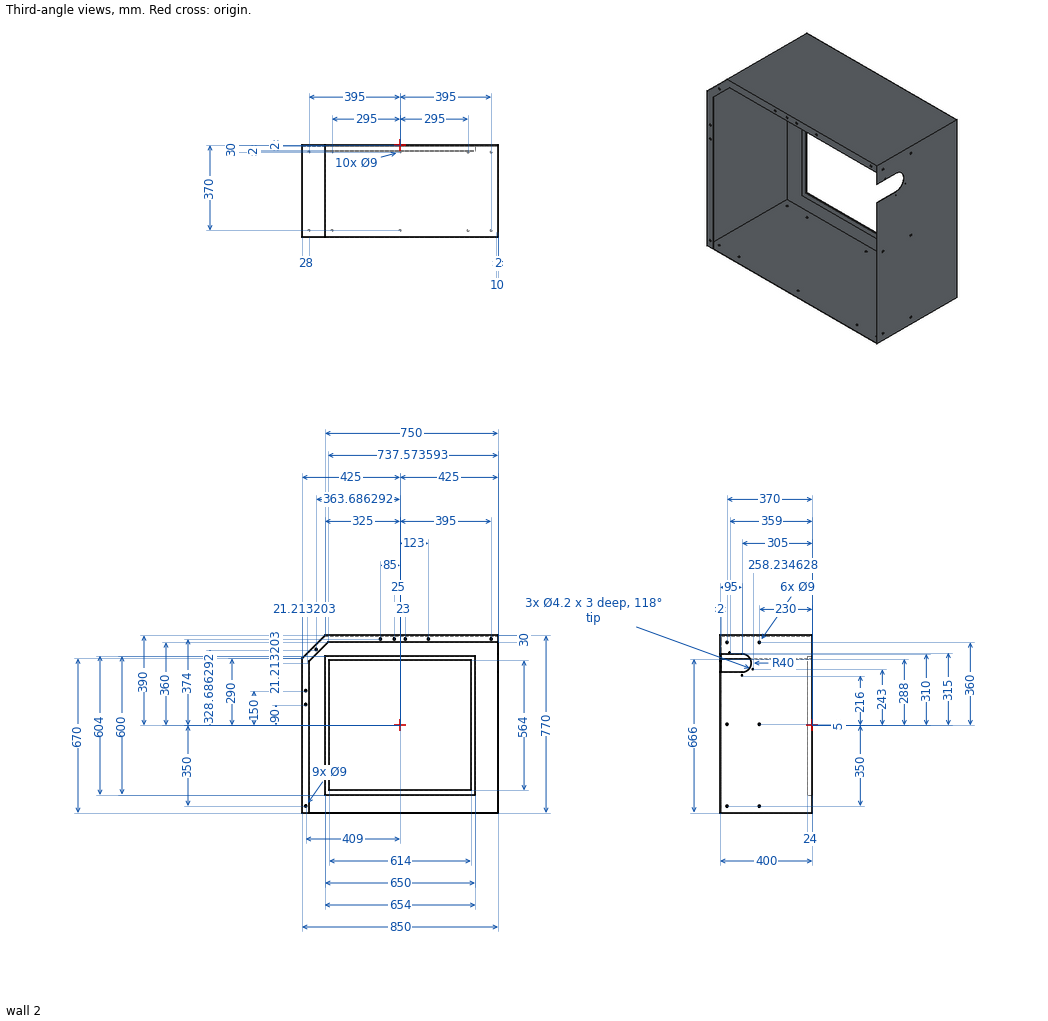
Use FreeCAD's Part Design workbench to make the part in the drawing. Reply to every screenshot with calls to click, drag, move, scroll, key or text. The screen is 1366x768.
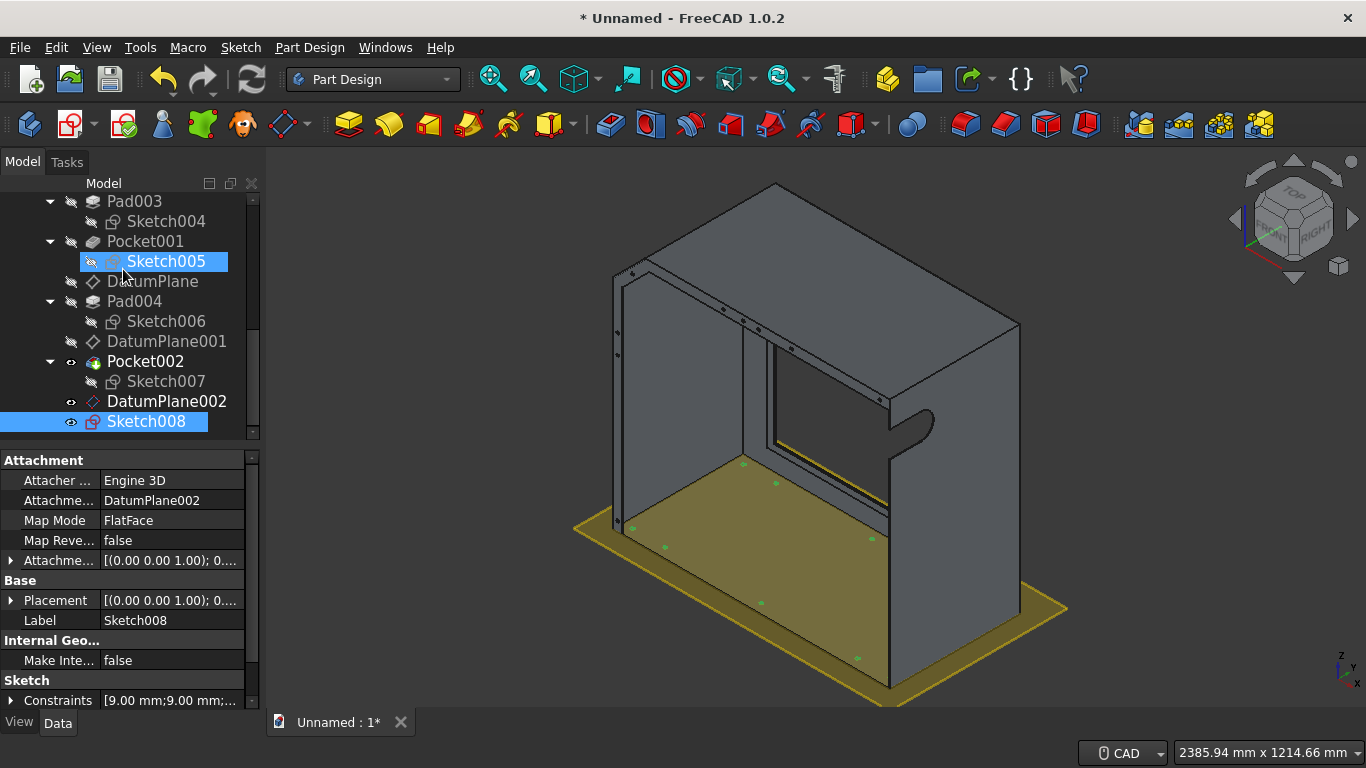
click(612, 124)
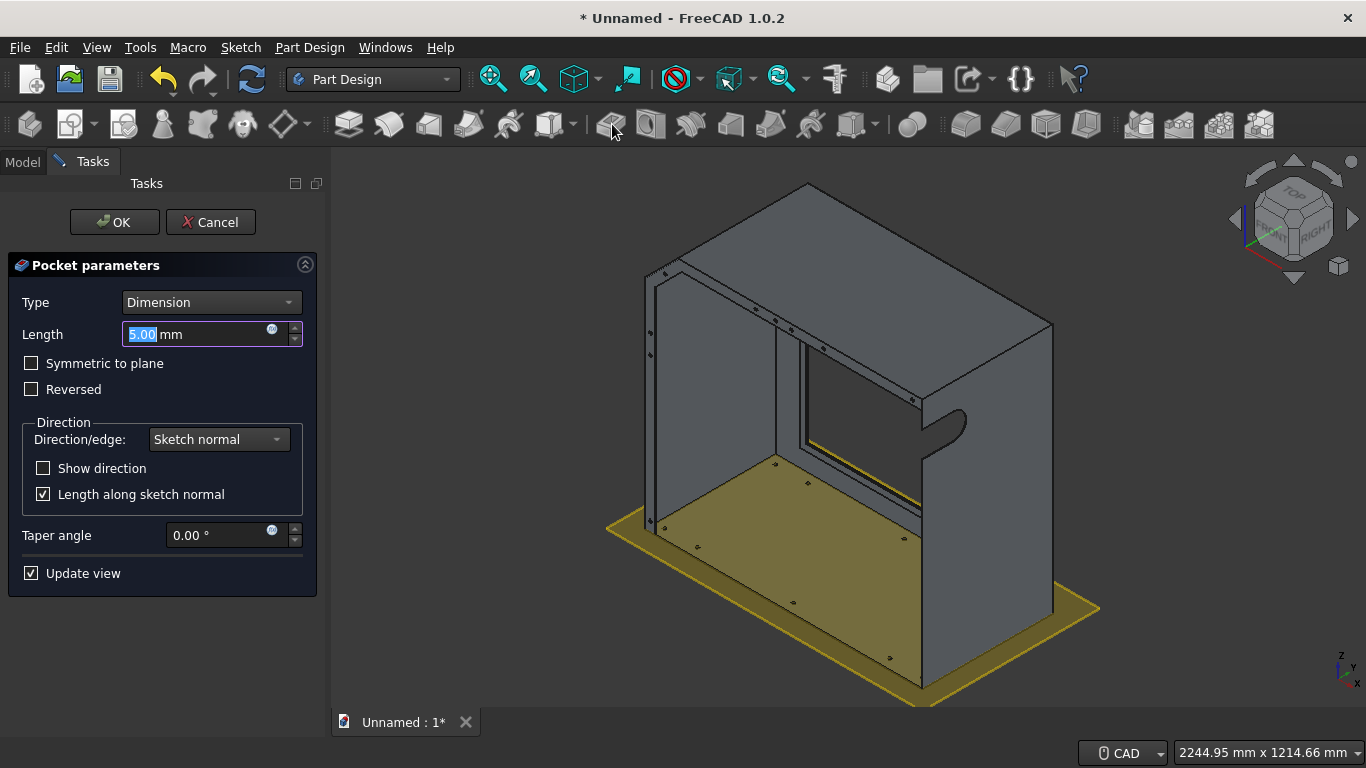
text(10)
key(Tab)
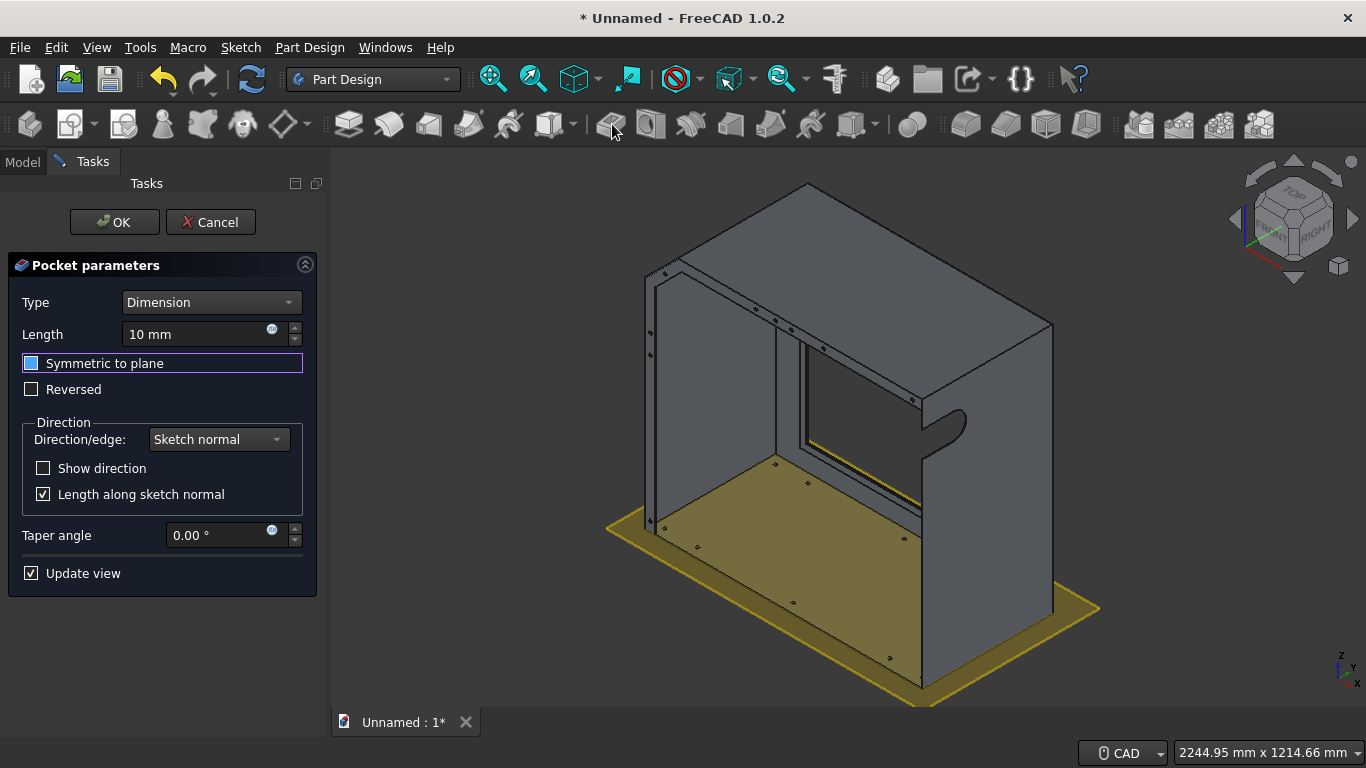
click(115, 222)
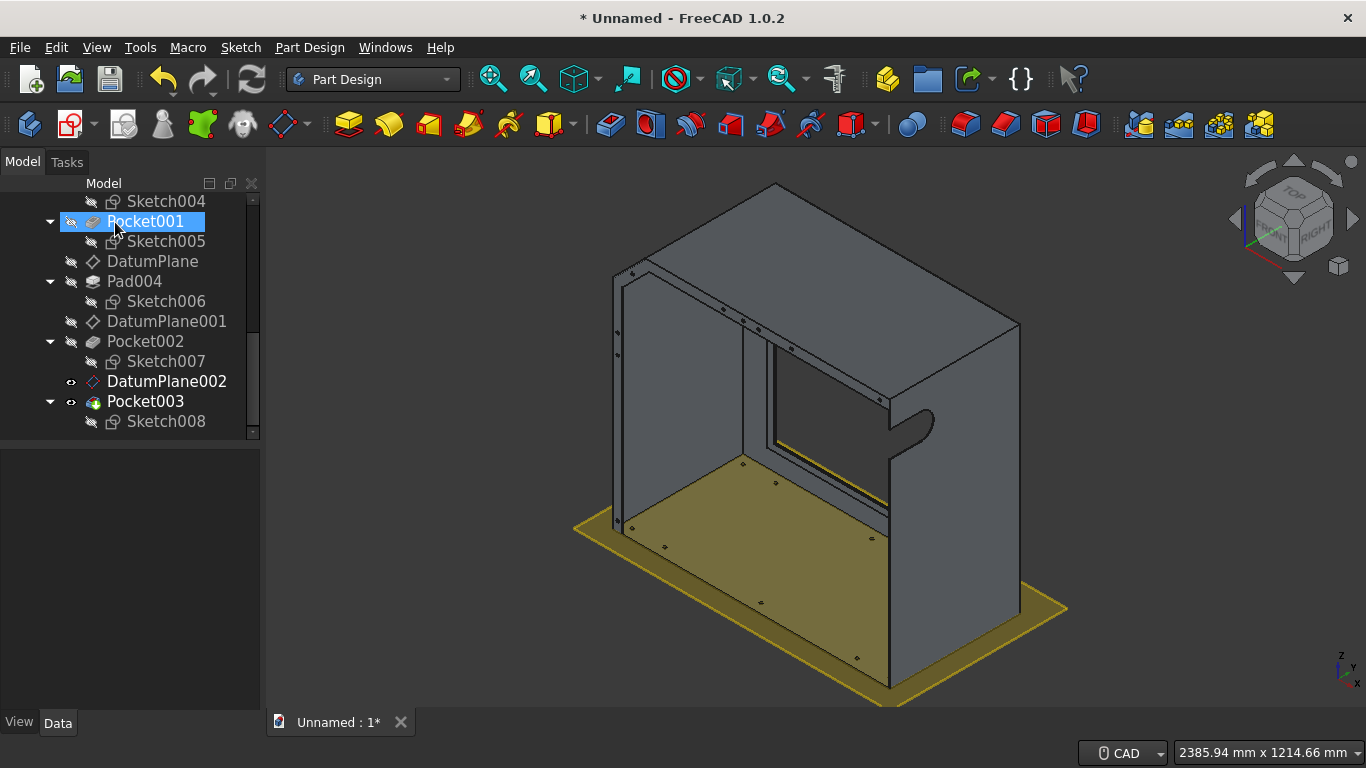
click(116, 382)
key(space)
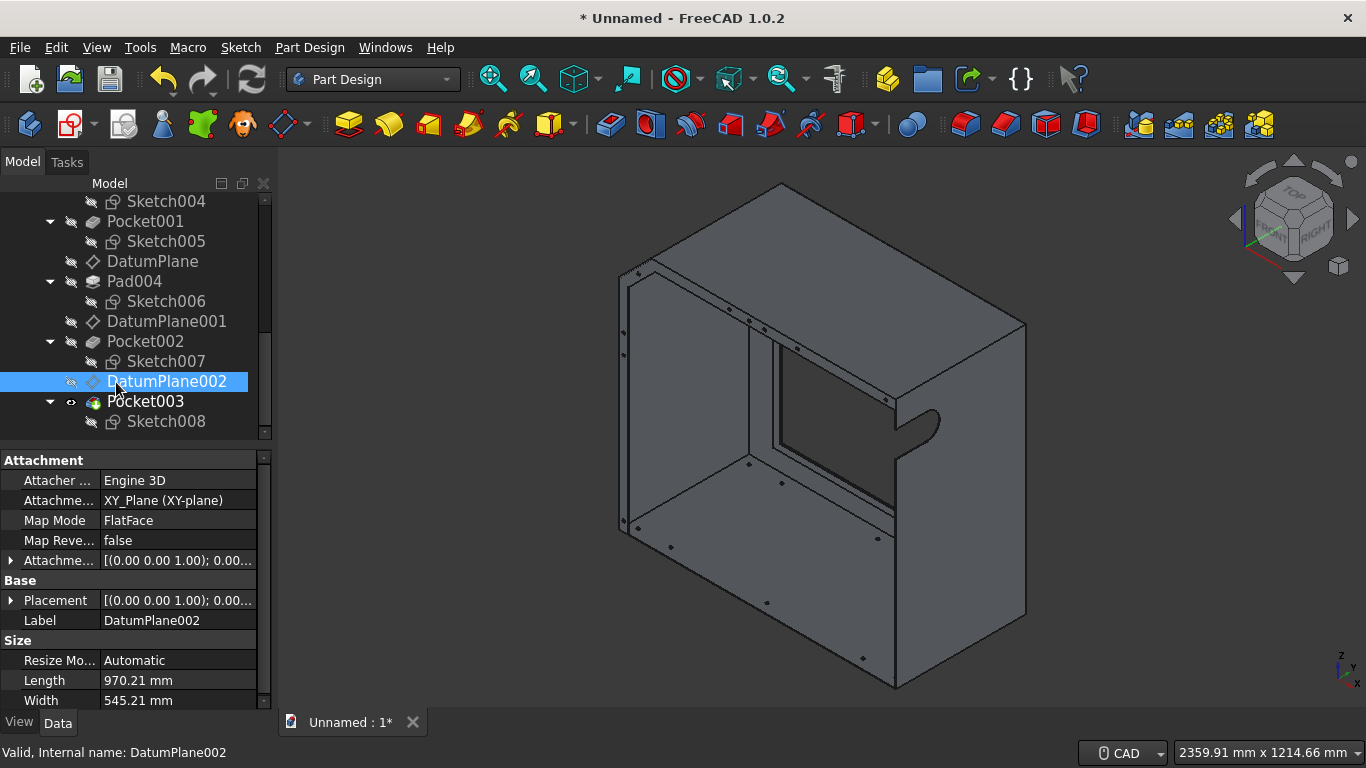
click(961, 506)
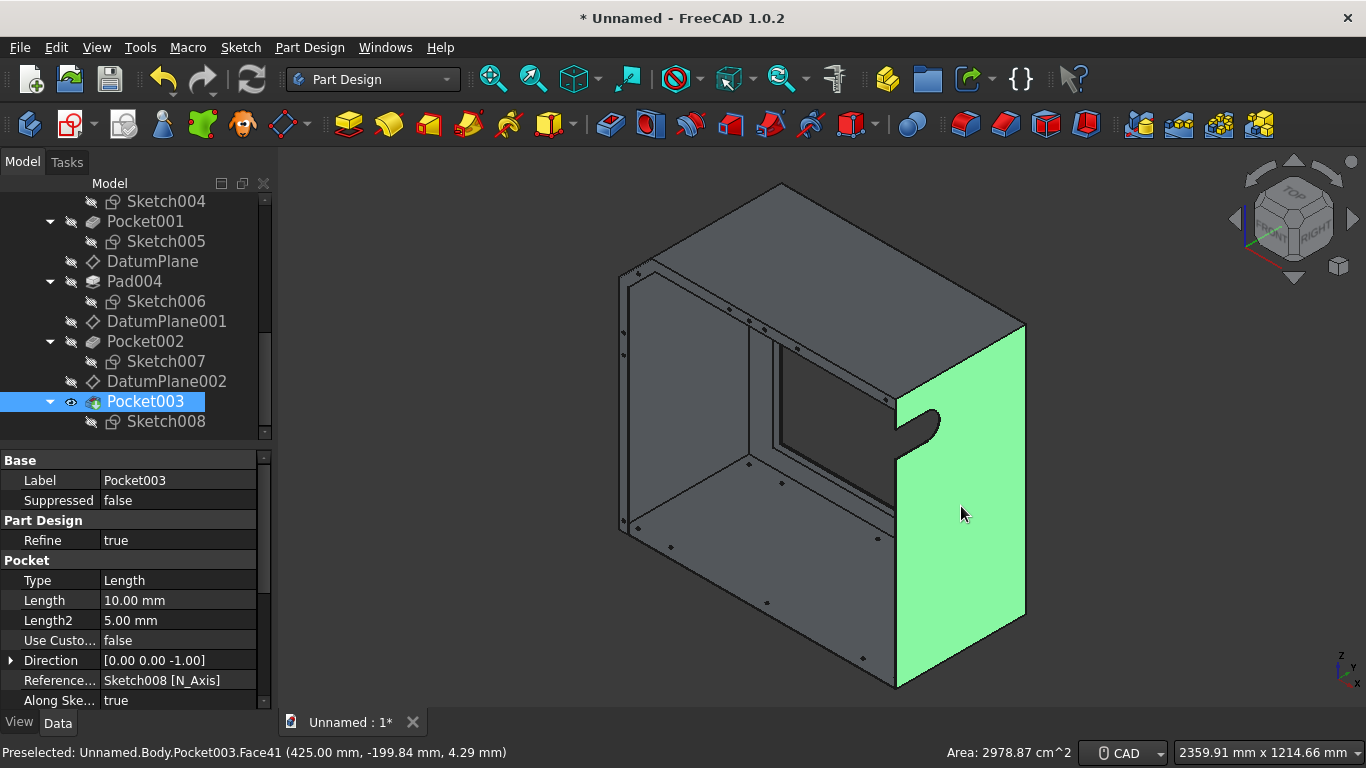
click(70, 124)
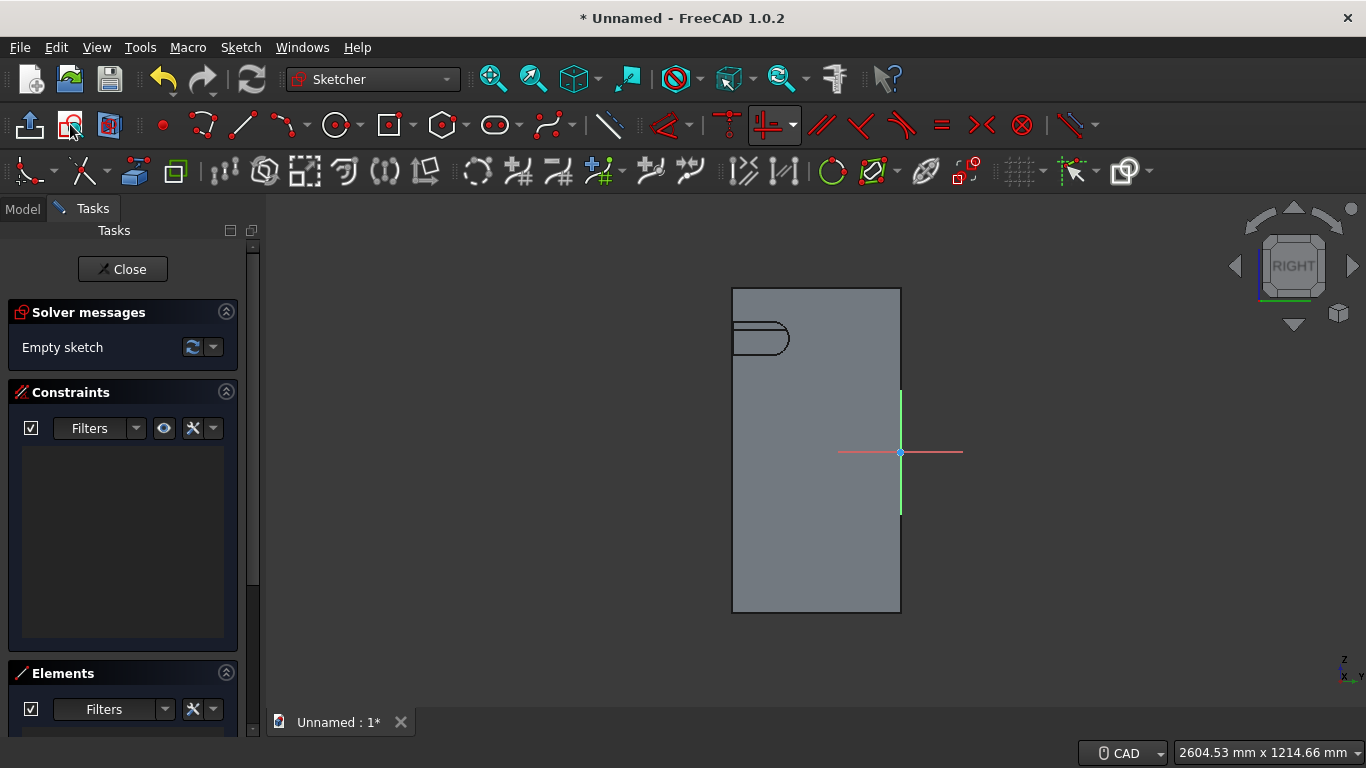
click(336, 126)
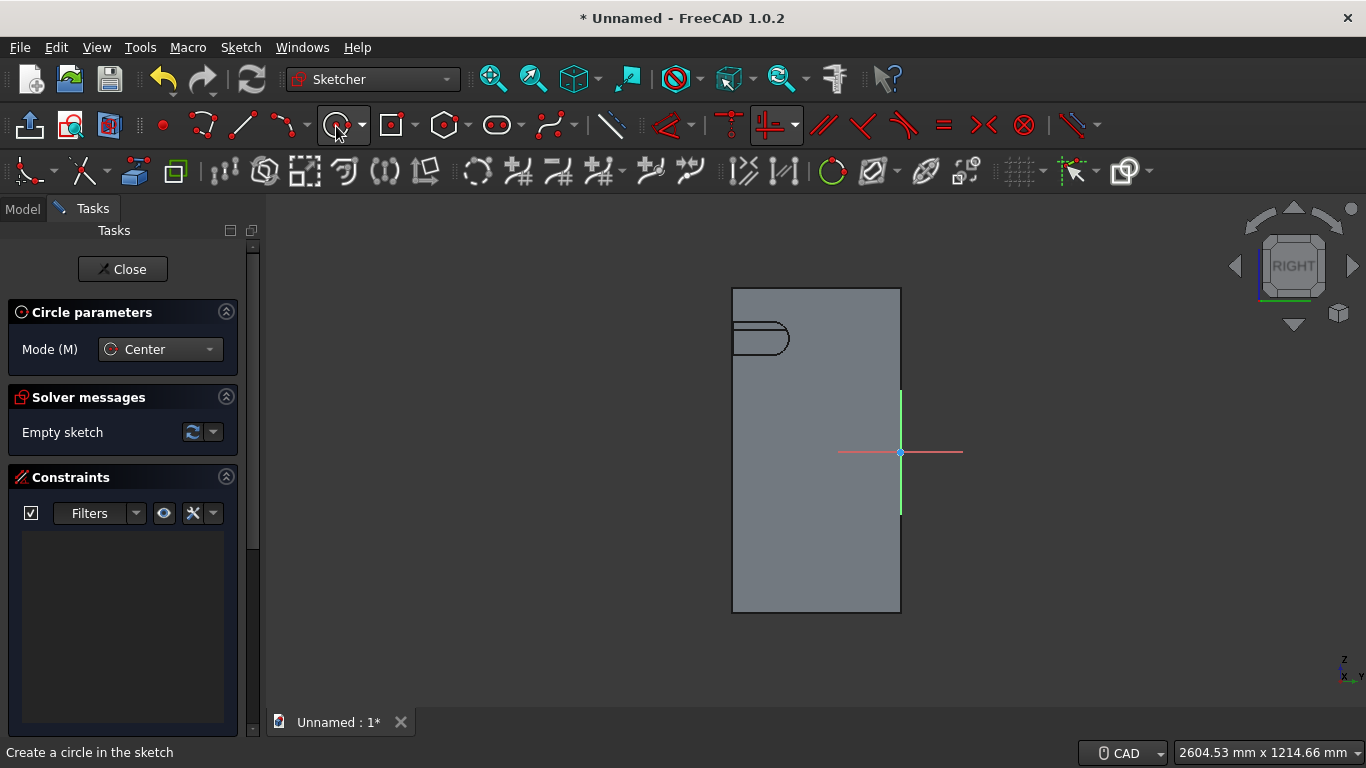
scroll(804, 300, up, 13)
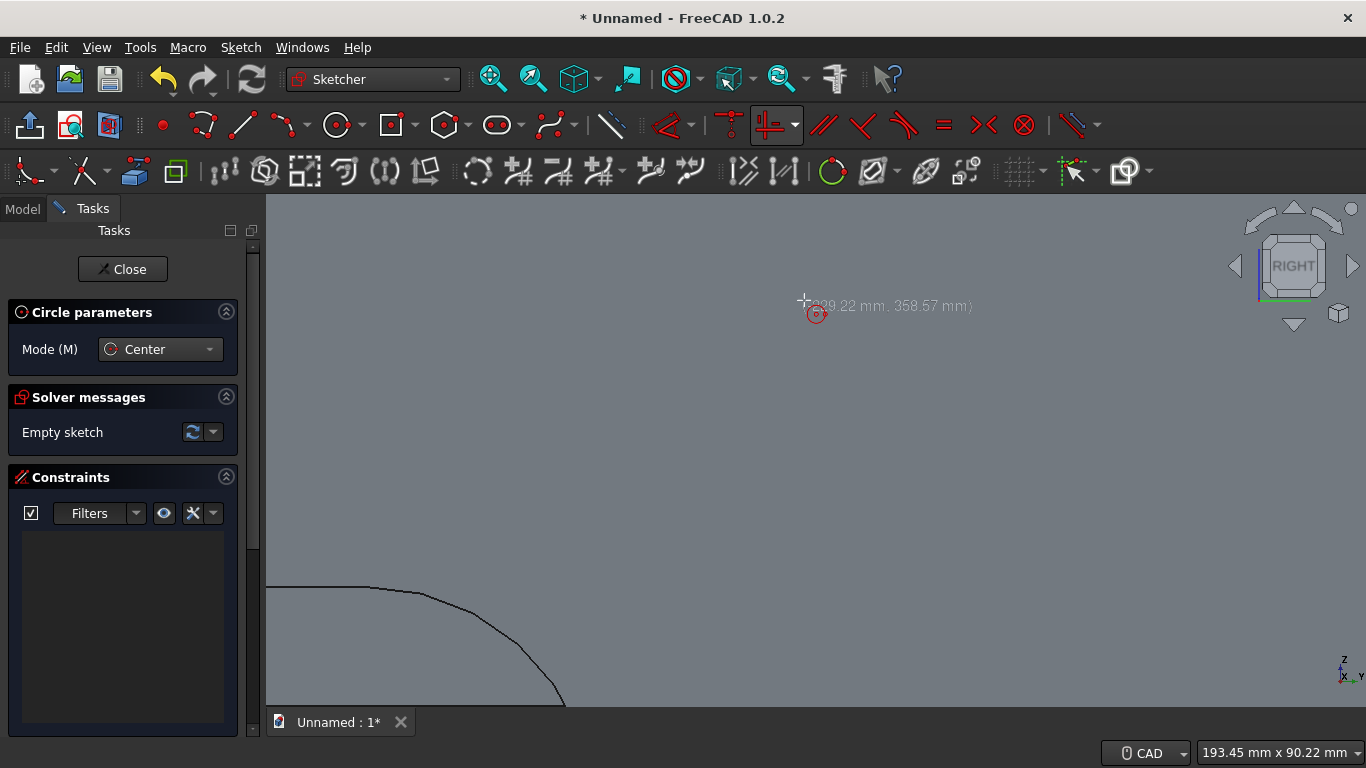
scroll(724, 300, down, 13)